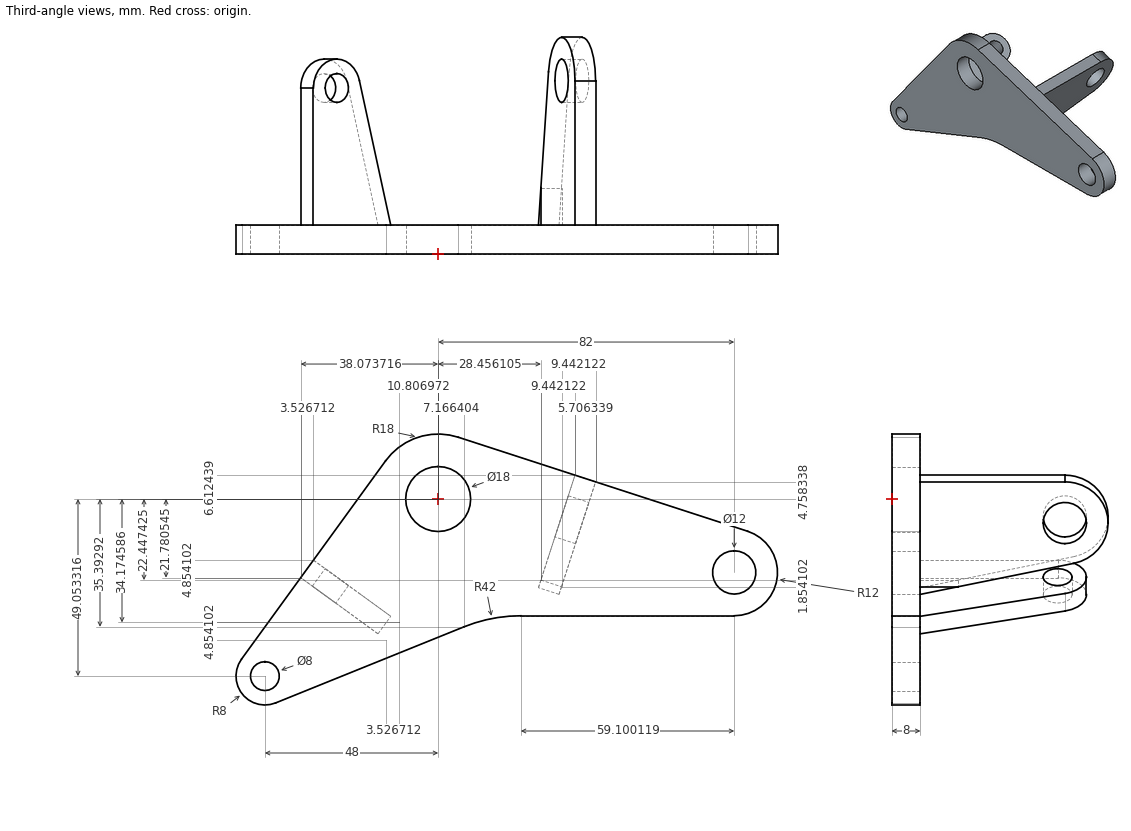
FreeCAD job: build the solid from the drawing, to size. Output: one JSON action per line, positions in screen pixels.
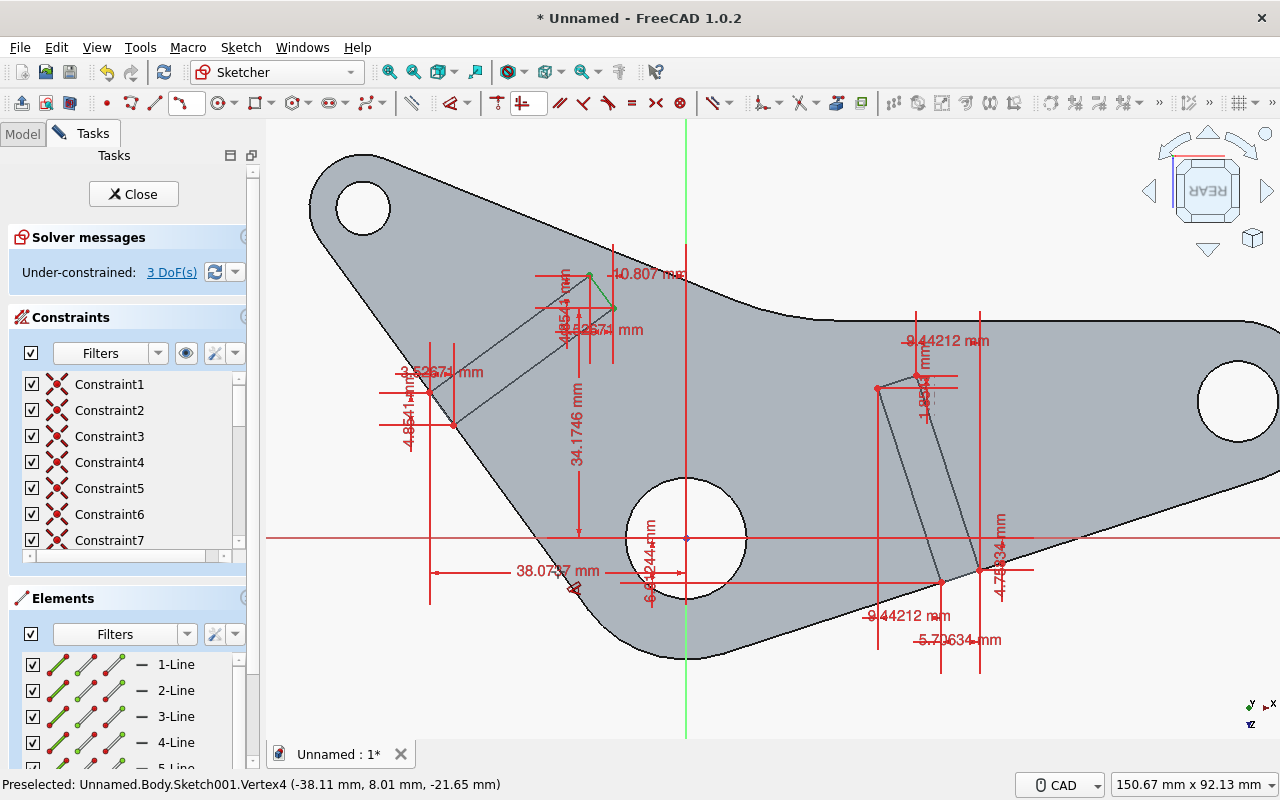
{"action": "left_click", "coordinate": [430, 393]}
{"action": "left_click", "coordinate": [396, 466]}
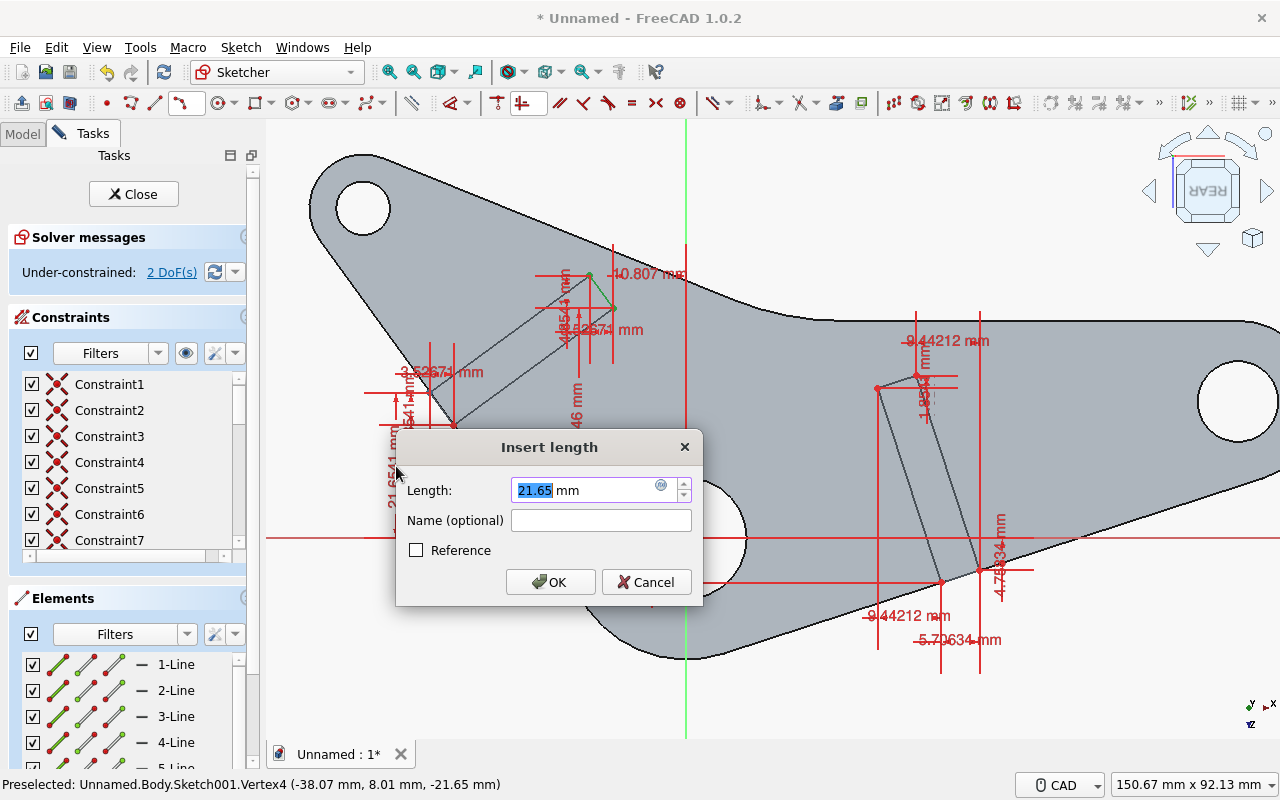
{"action": "type", "text": "21.780545"}
{"action": "key", "text": "Return"}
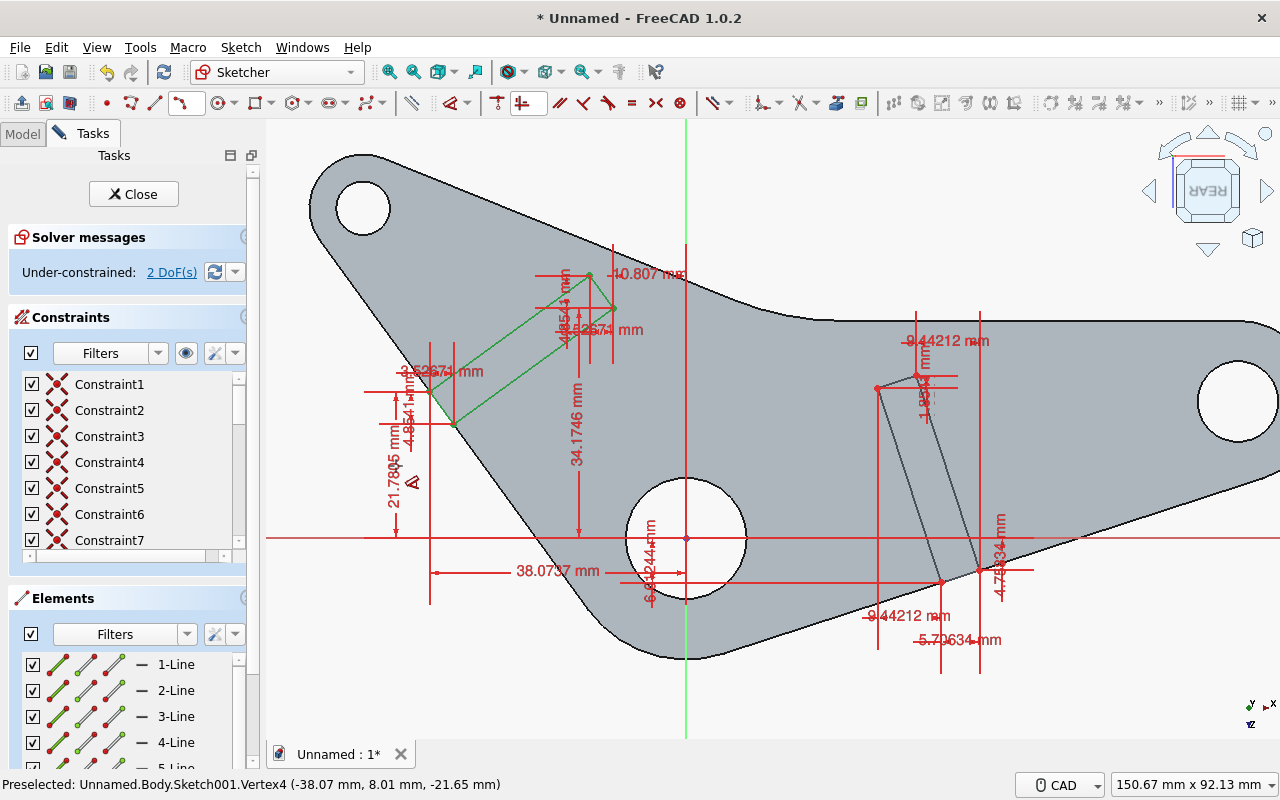
{"action": "left_click", "coordinate": [878, 388]}
{"action": "left_click", "coordinate": [782, 572]}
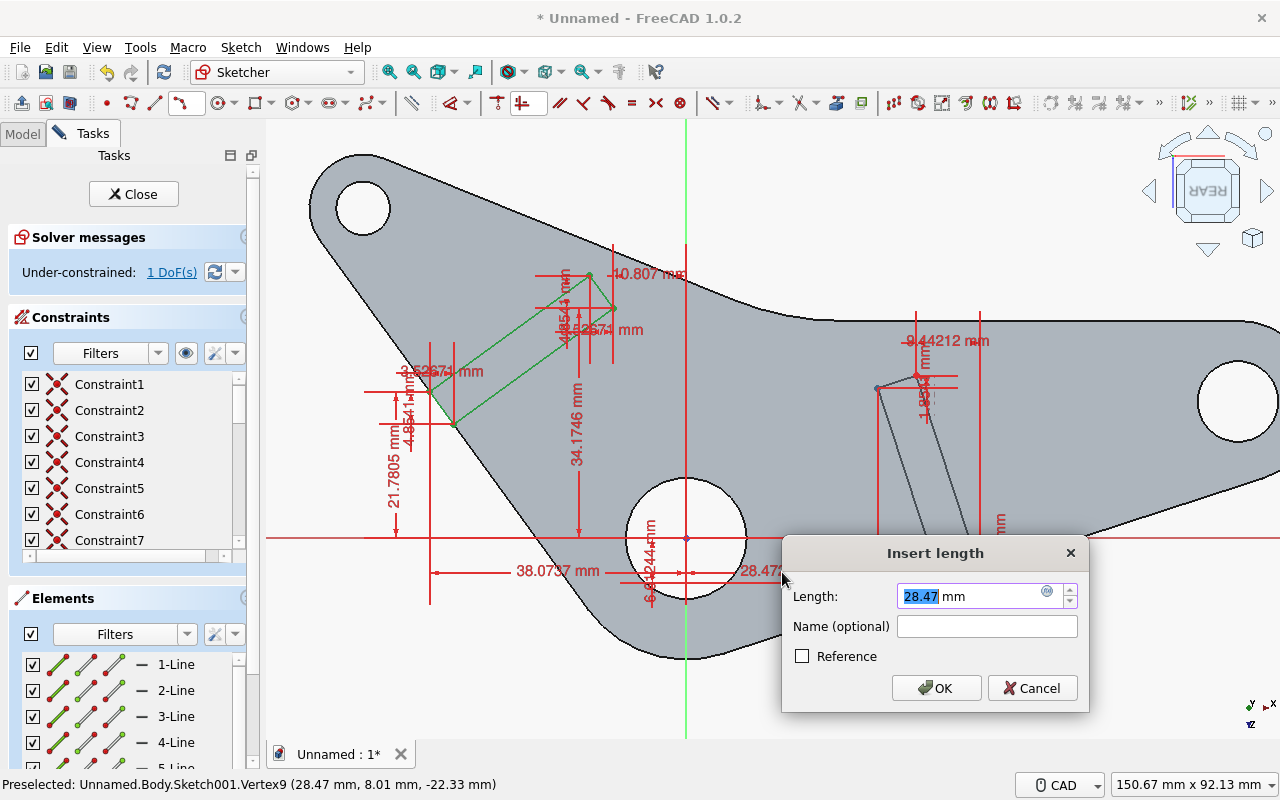
{"action": "type", "text": "28.456105"}
{"action": "key", "text": "Return"}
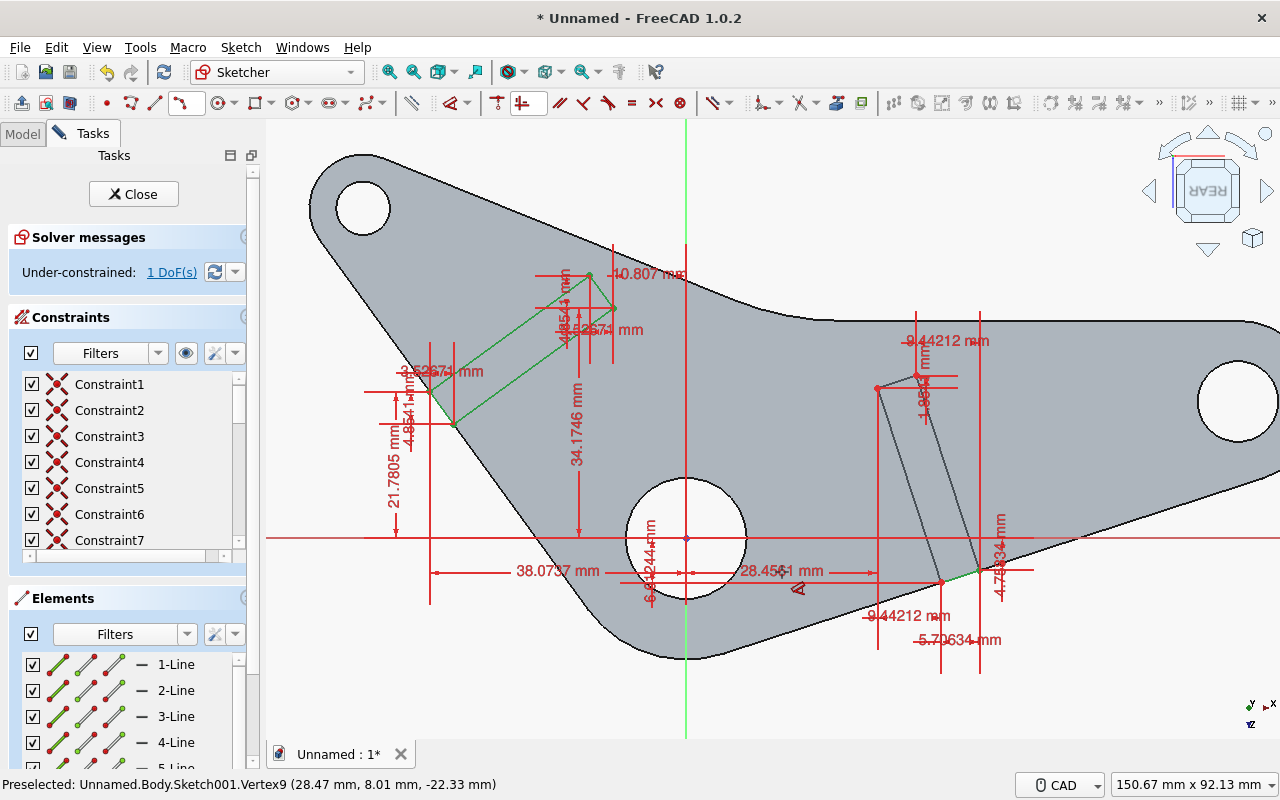
{"action": "left_click", "coordinate": [878, 388]}
{"action": "left_click", "coordinate": [912, 429]}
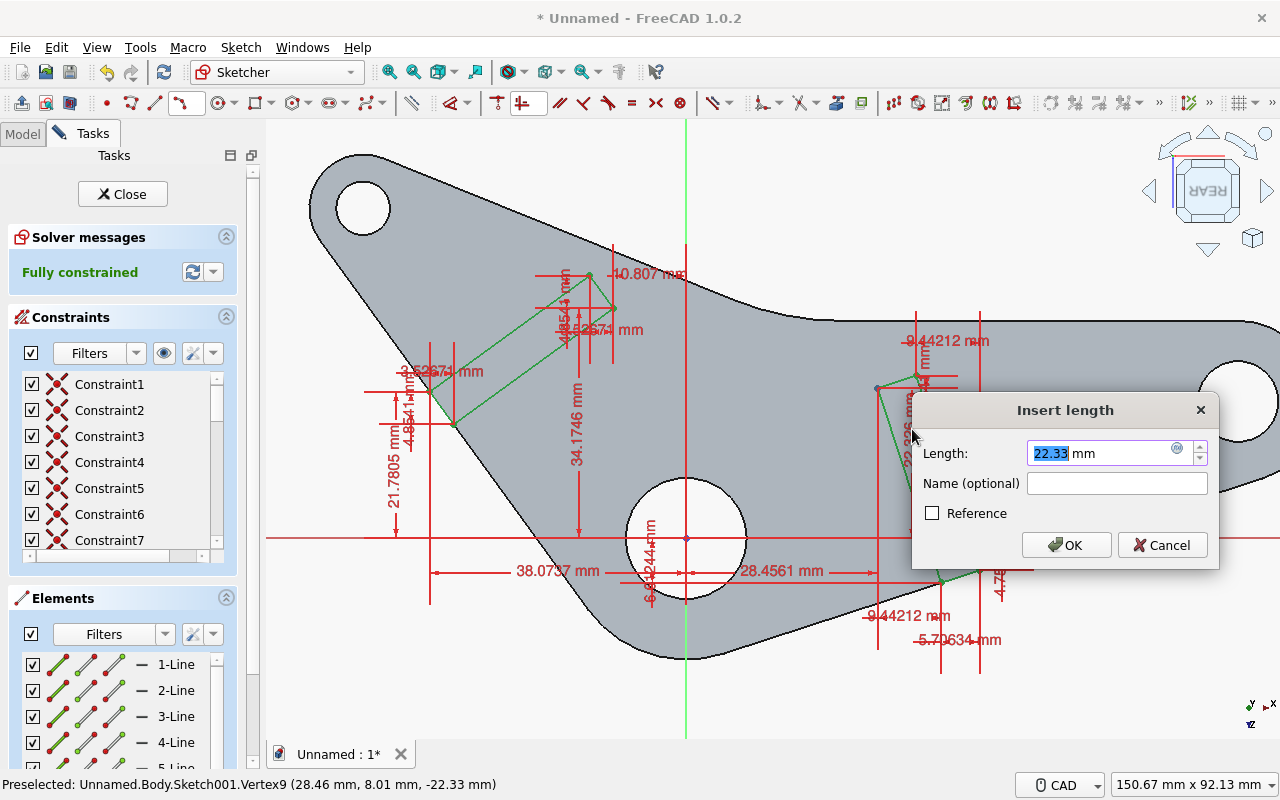
{"action": "type", "text": "22.447425"}
{"action": "key", "text": "Return"}
{"action": "key", "text": "Escape"}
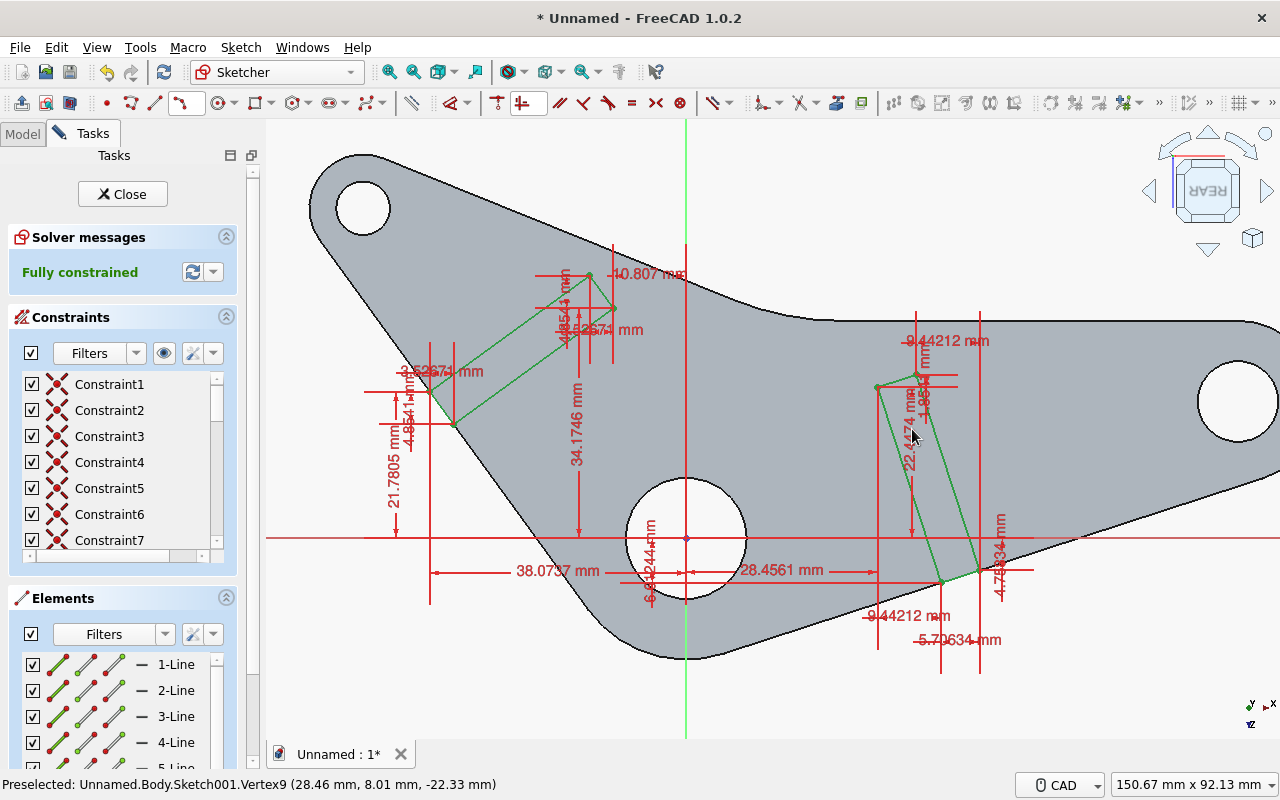
{"action": "left_click", "coordinate": [123, 194]}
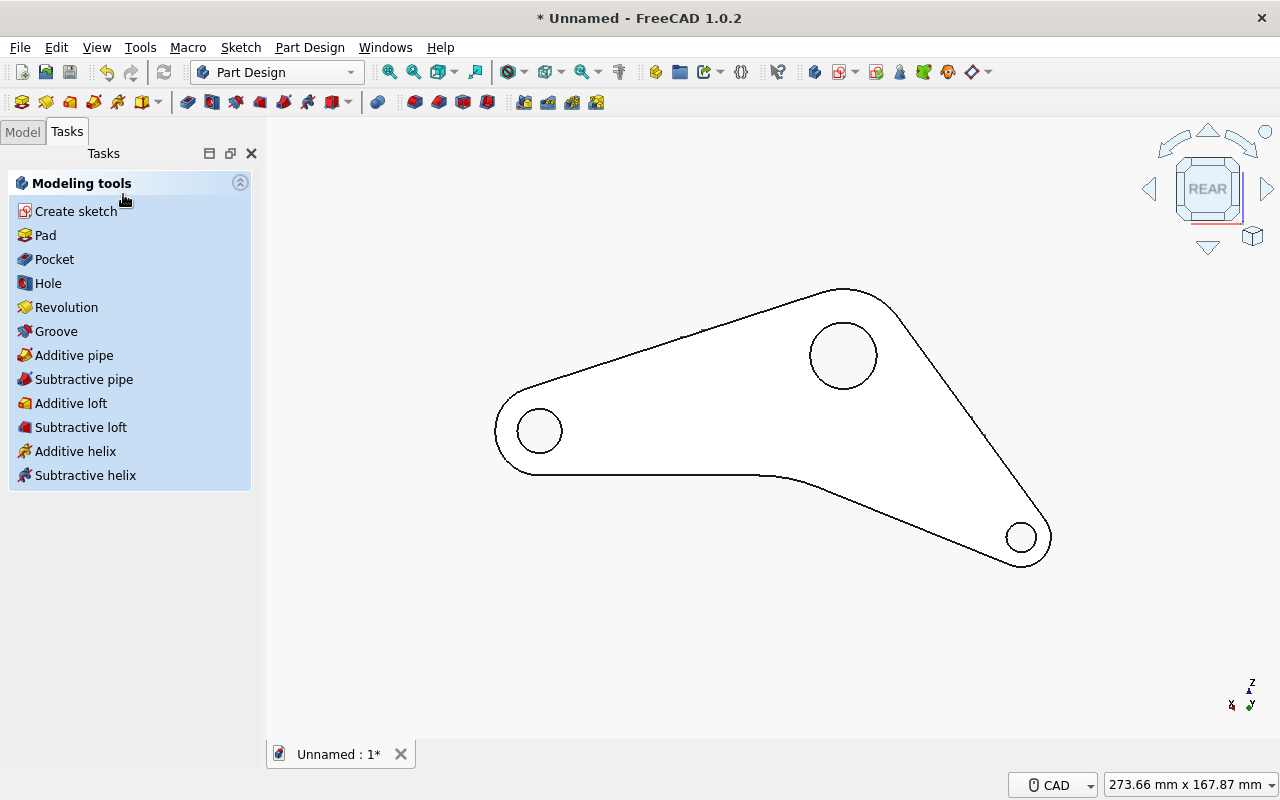
{"action": "left_click", "coordinate": [22, 102]}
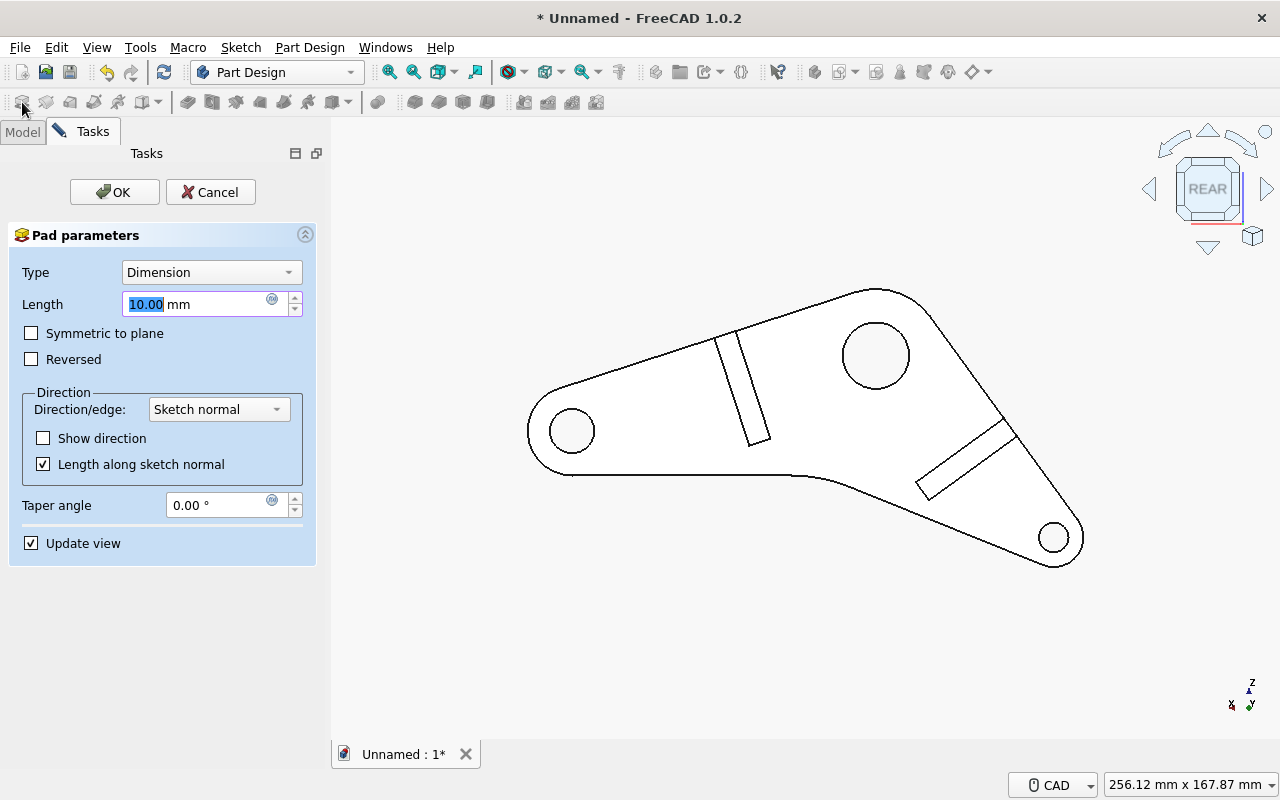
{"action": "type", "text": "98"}
{"action": "key", "text": "Tab"}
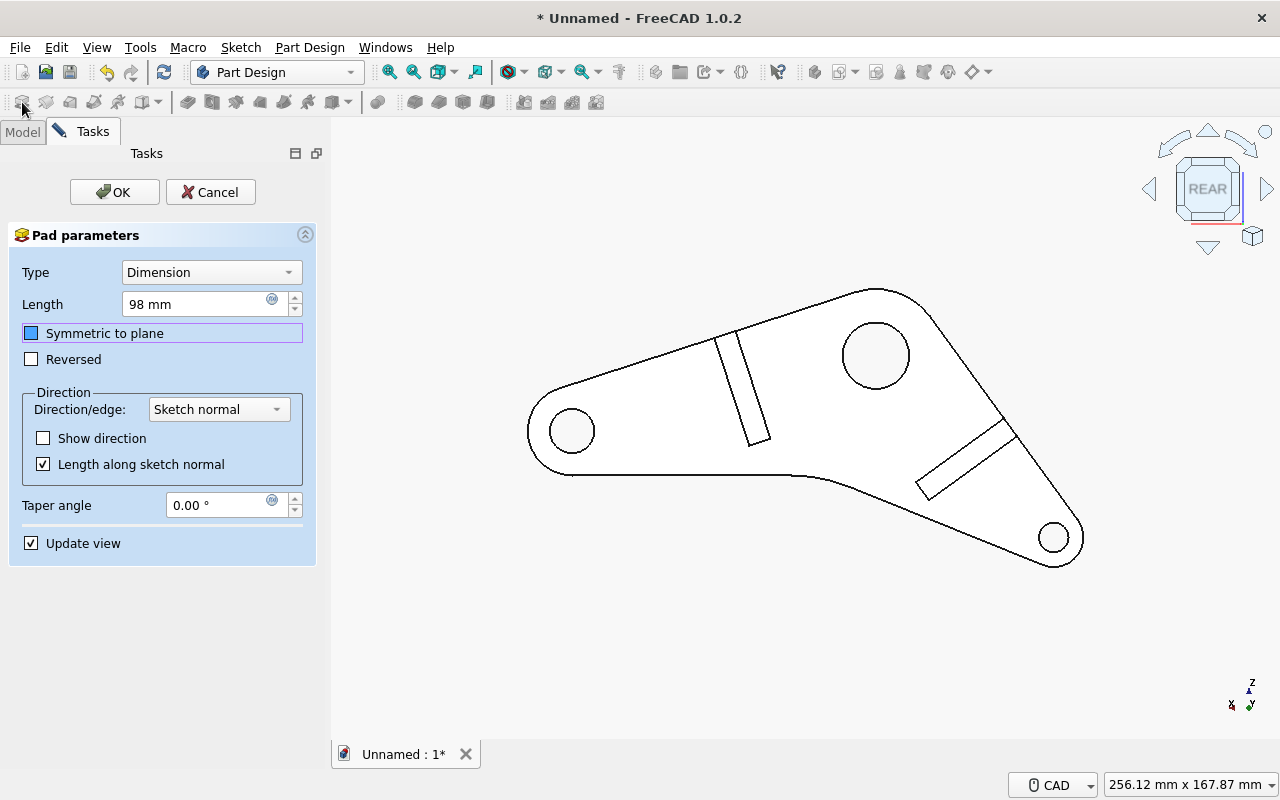
{"action": "left_click", "coordinate": [115, 192]}